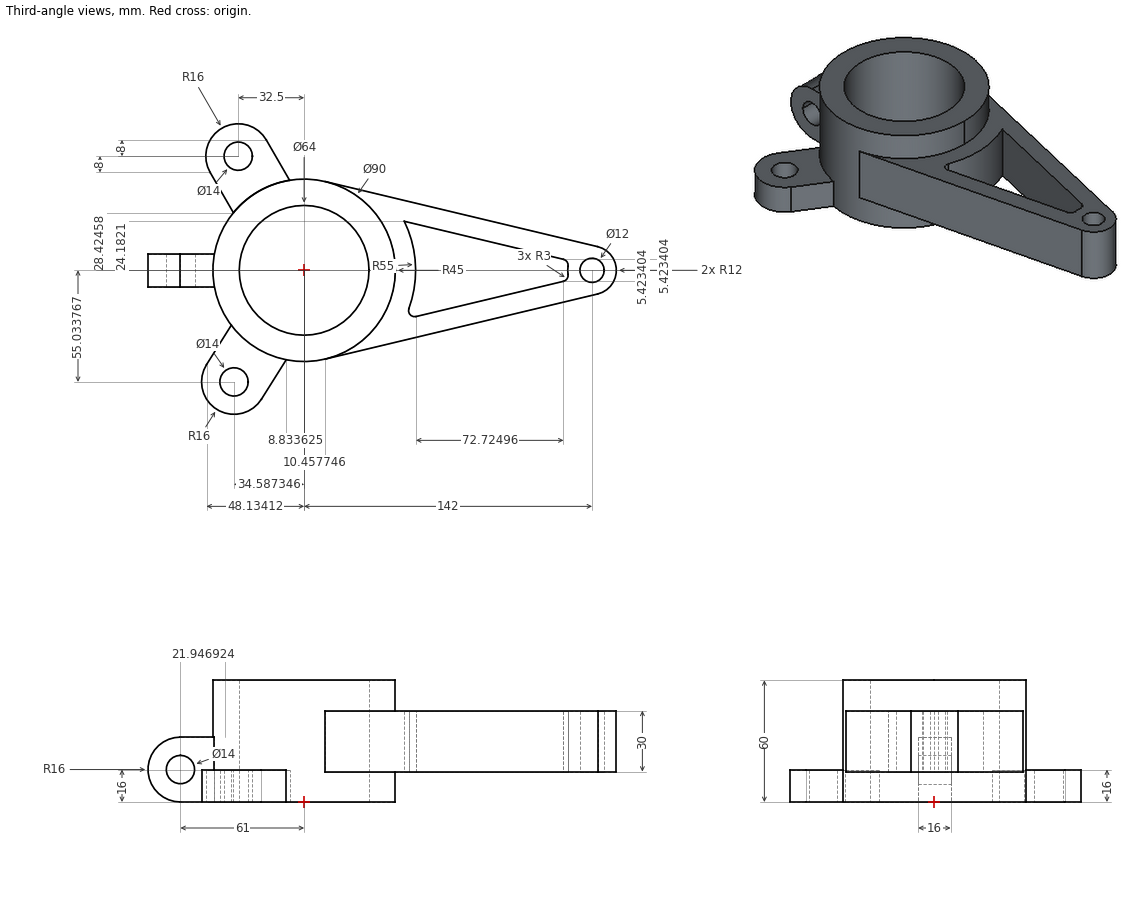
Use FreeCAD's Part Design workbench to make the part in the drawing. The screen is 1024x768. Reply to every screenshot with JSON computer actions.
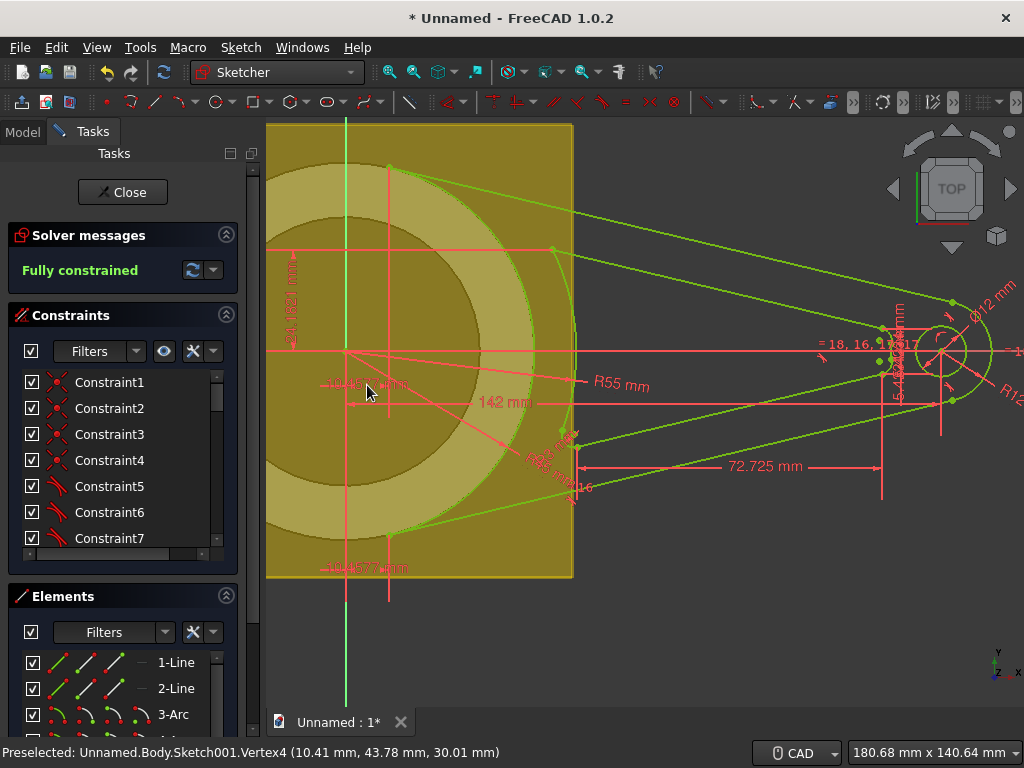
{"action": "left_click", "coordinate": [123, 192]}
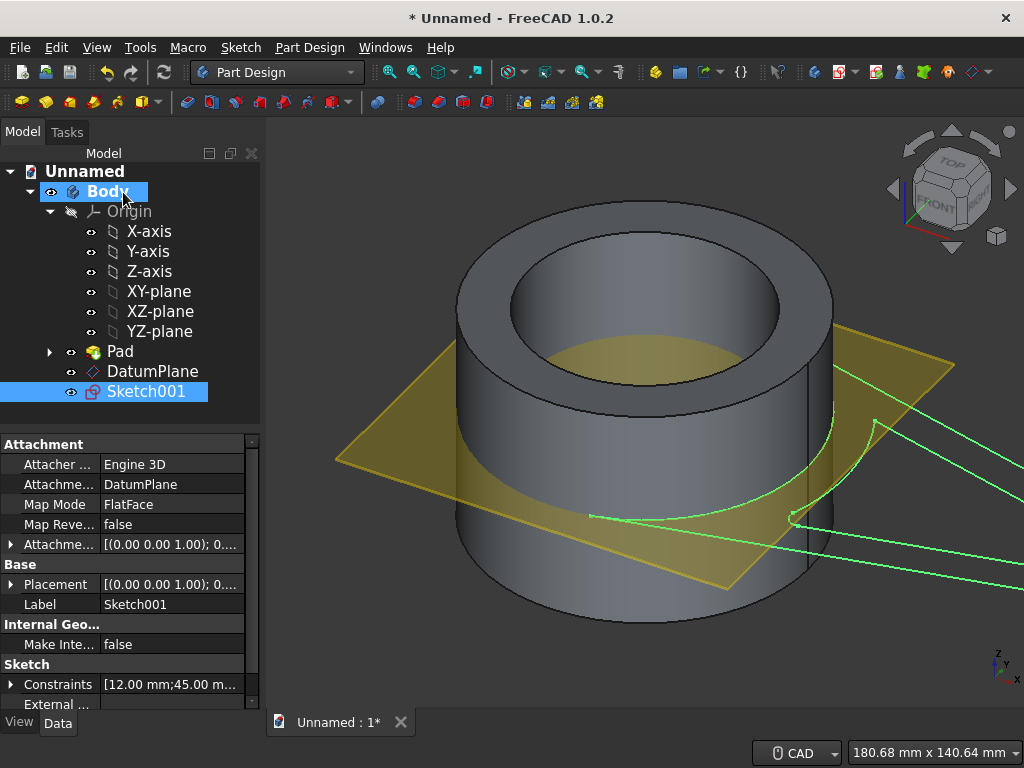
{"action": "left_click", "coordinate": [22, 102]}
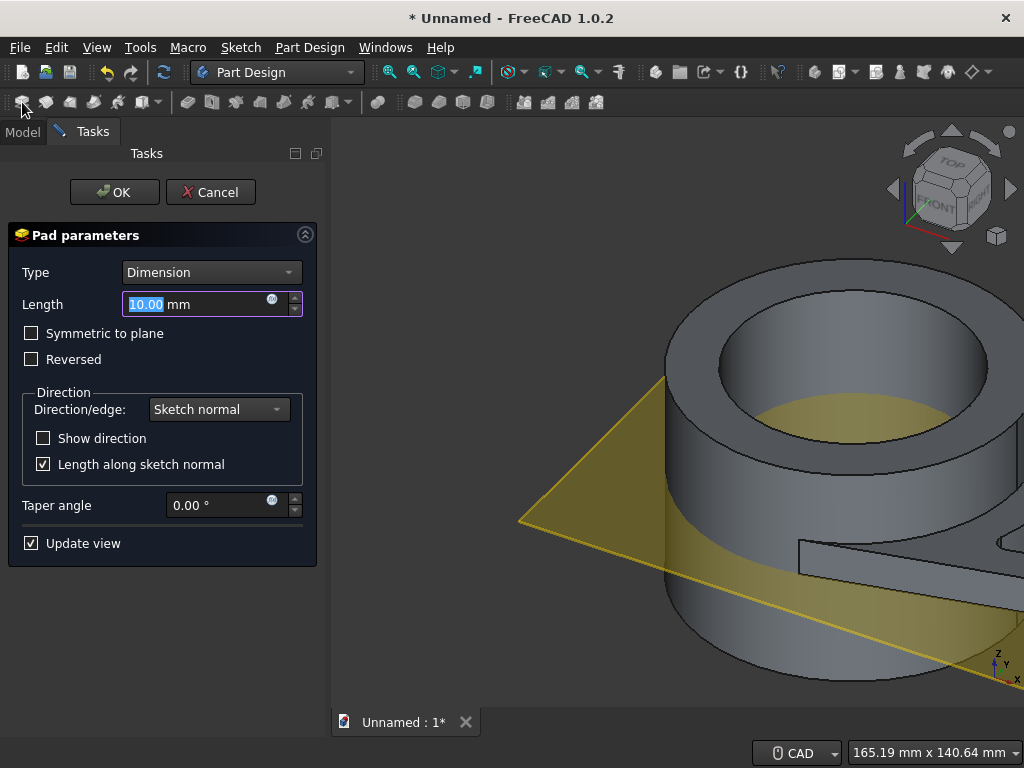
{"action": "type", "text": "30"}
{"action": "key", "text": "Tab"}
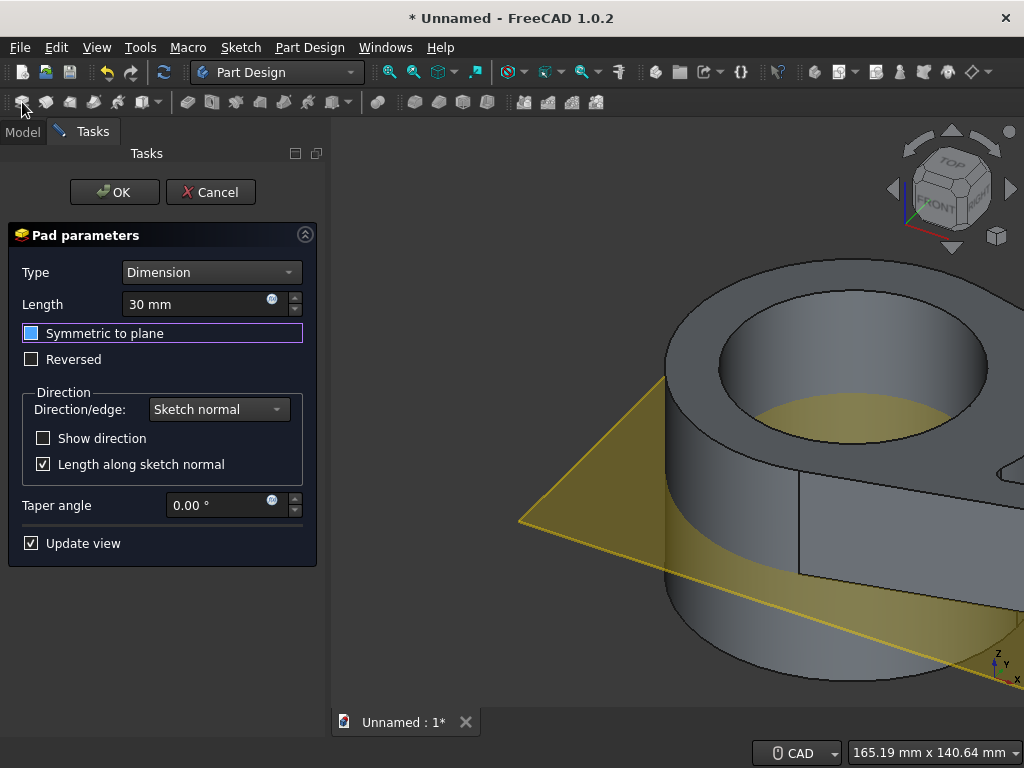
{"action": "left_click", "coordinate": [30, 333]}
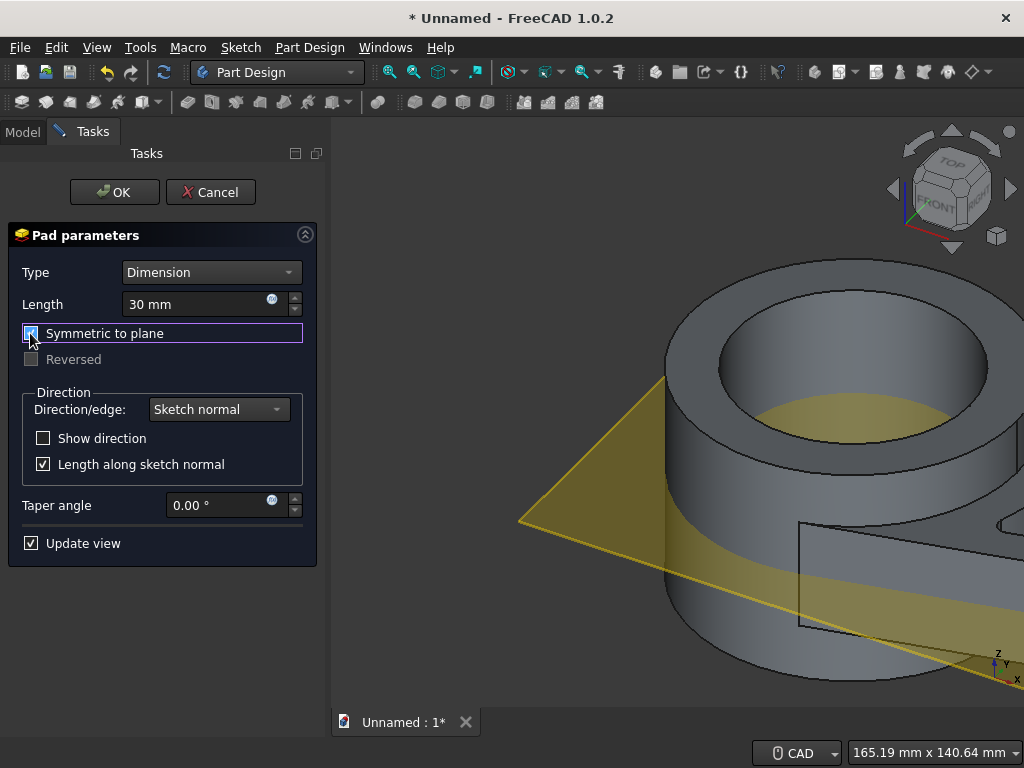
{"action": "left_click", "coordinate": [115, 192]}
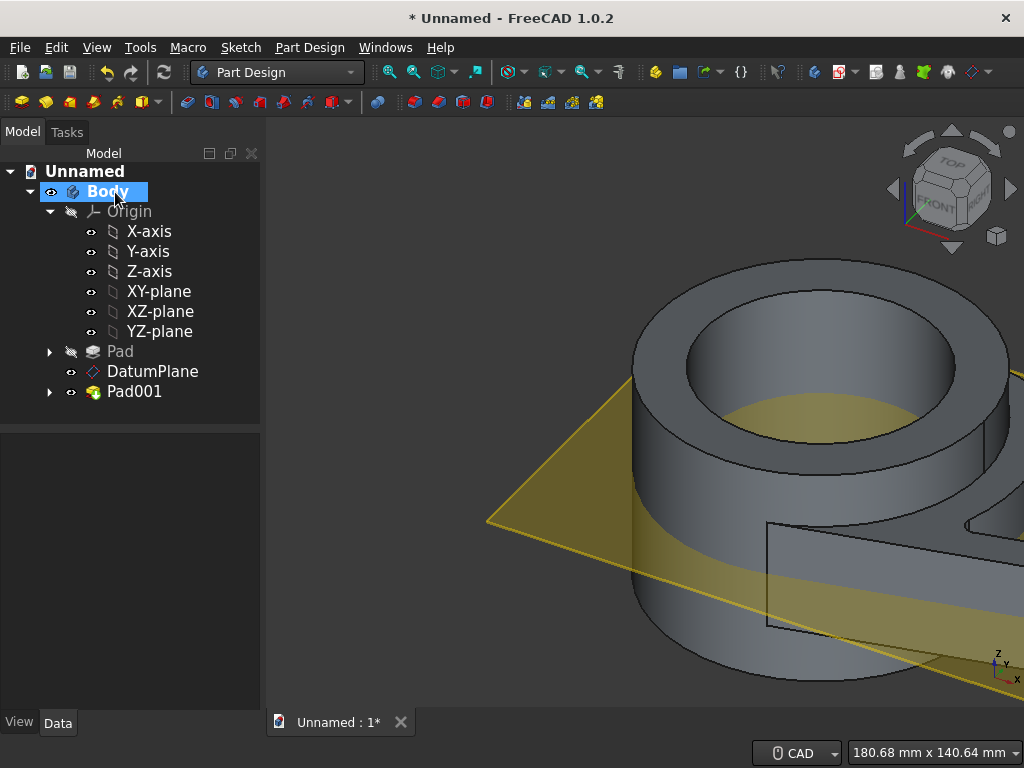
{"action": "left_click", "coordinate": [116, 372]}
{"action": "key", "text": "space"}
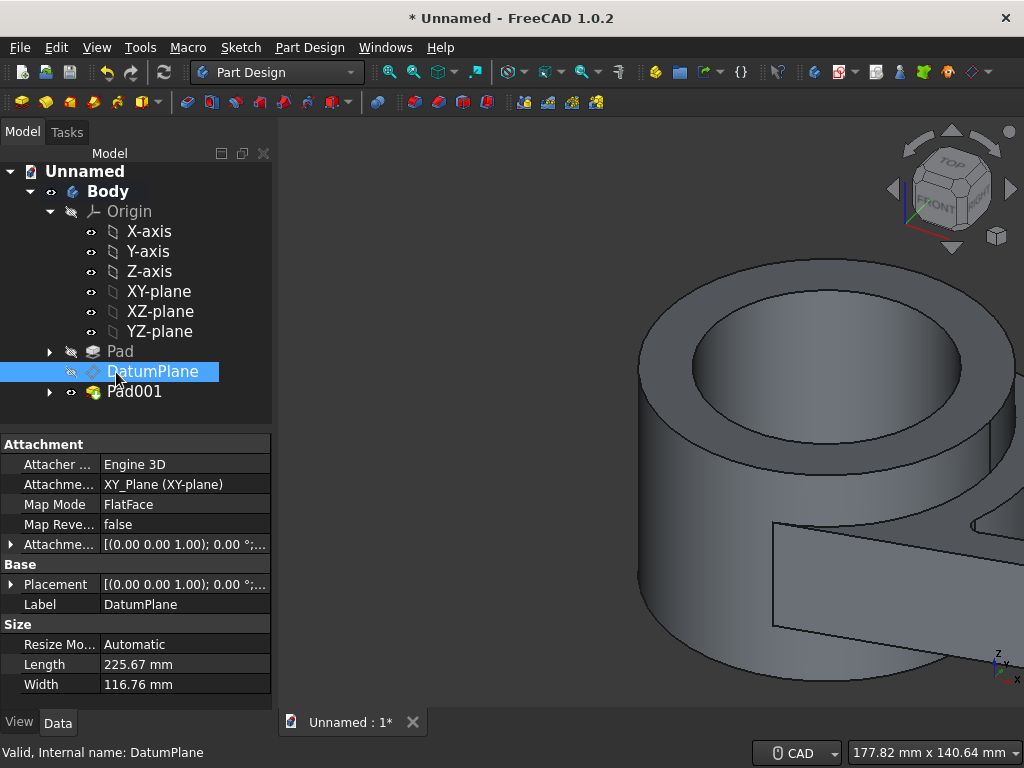
{"action": "left_click", "coordinate": [390, 72]}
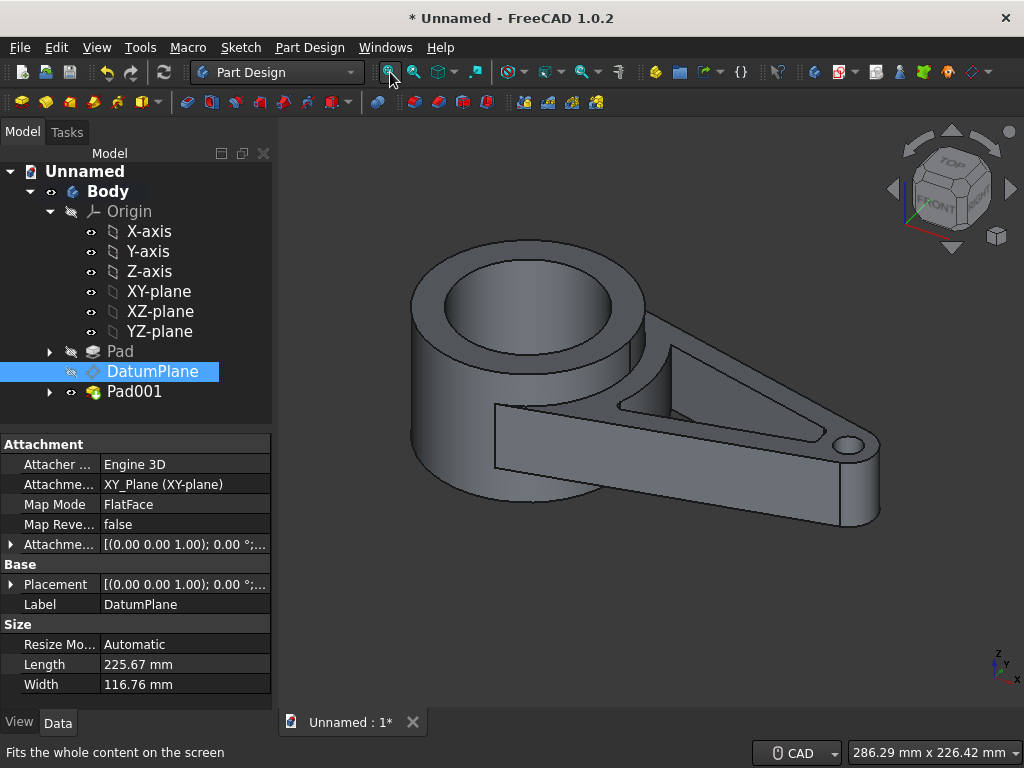
{"action": "left_click", "coordinate": [318, 667]}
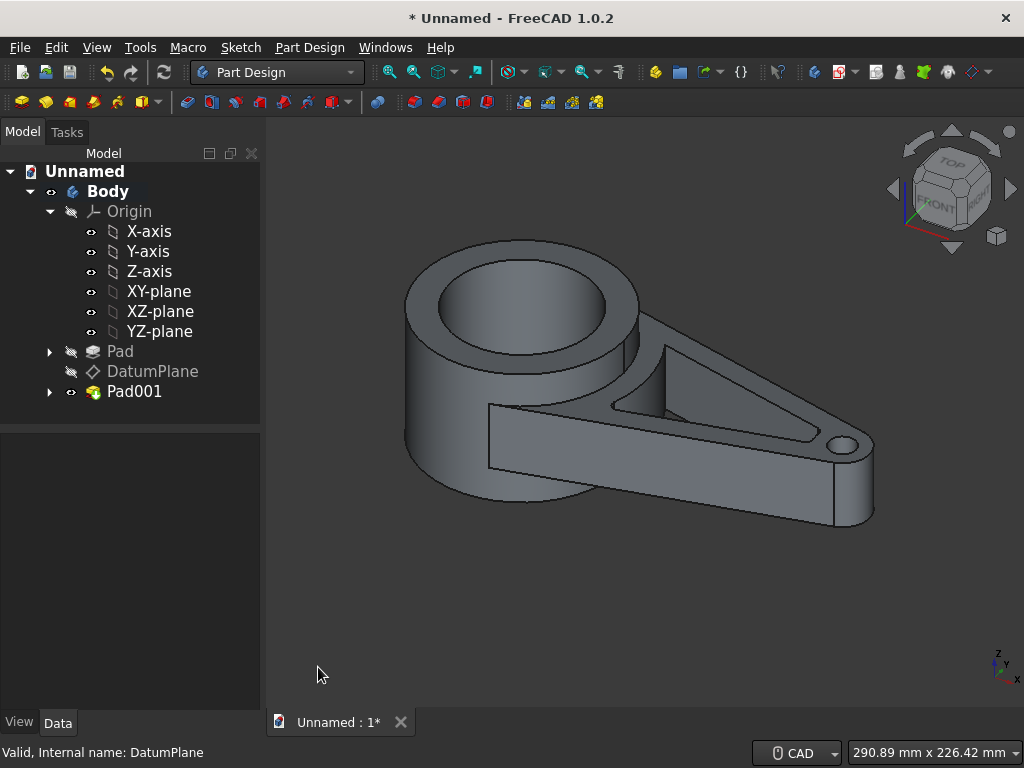
{"action": "left_click", "coordinate": [840, 72]}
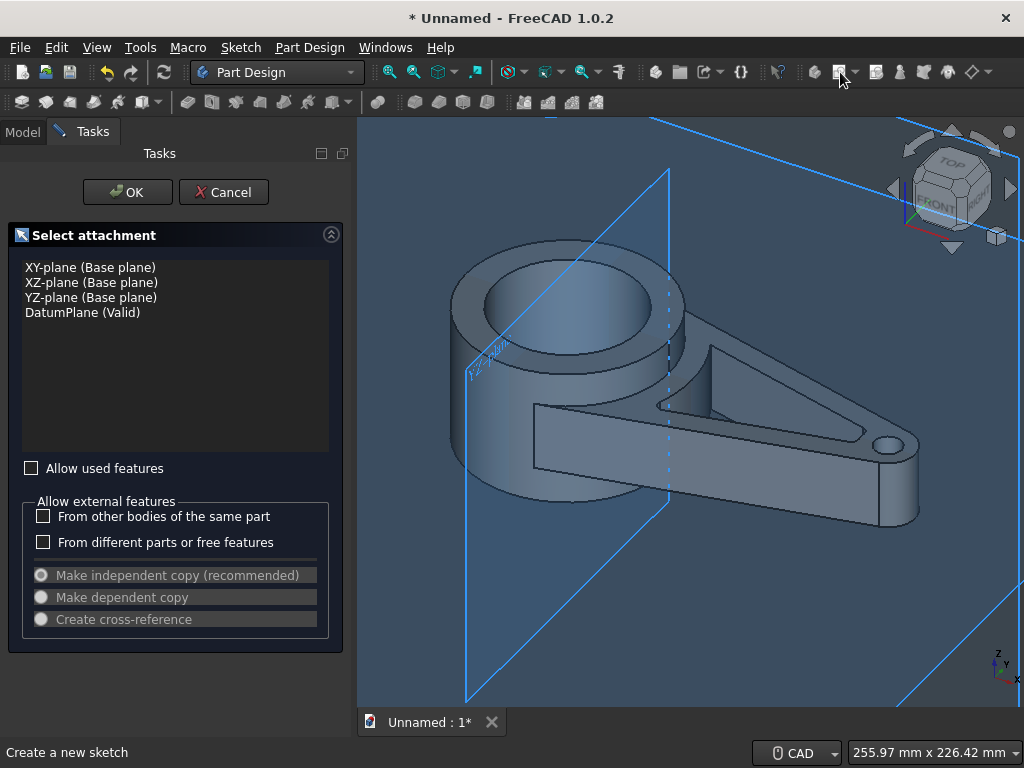
{"action": "left_click", "coordinate": [82, 268]}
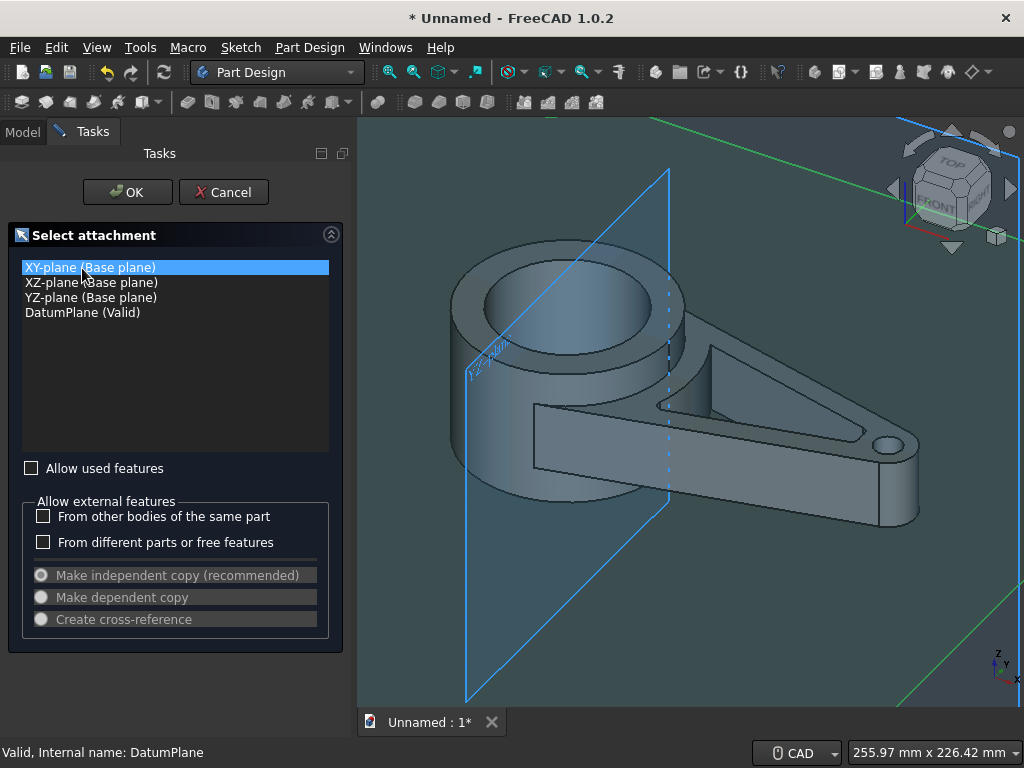
{"action": "left_click", "coordinate": [128, 192]}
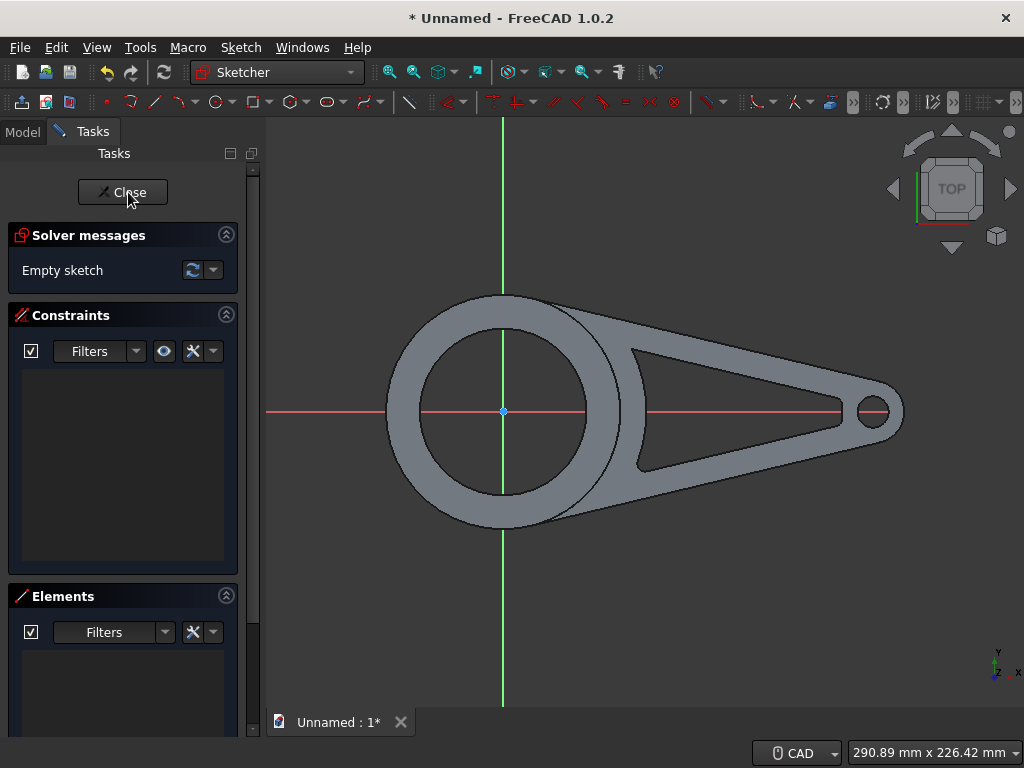
{"action": "key", "text": "q s"}